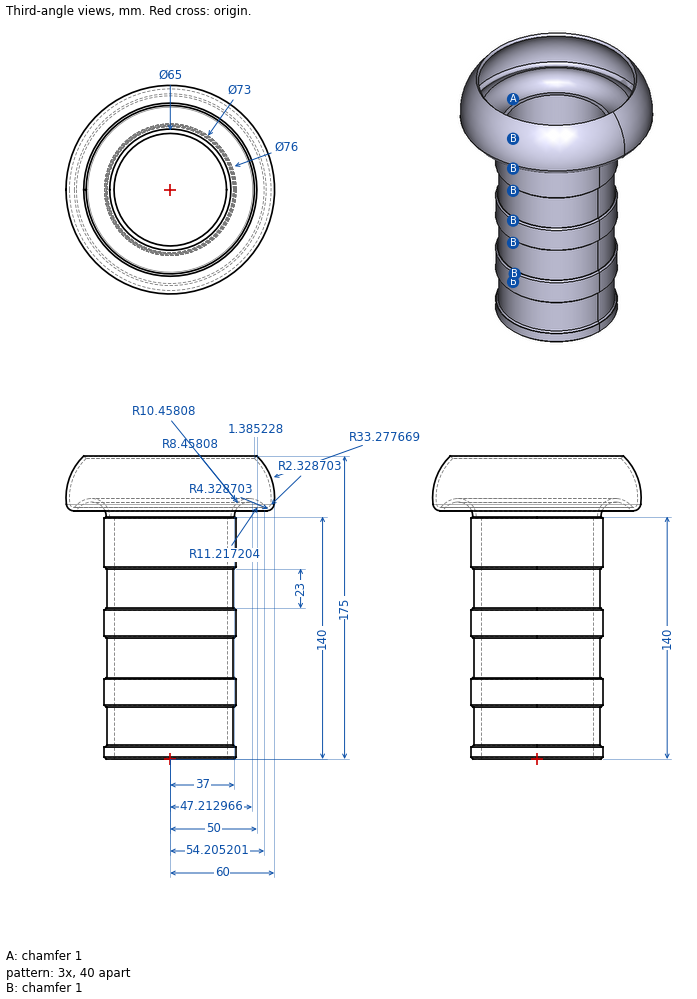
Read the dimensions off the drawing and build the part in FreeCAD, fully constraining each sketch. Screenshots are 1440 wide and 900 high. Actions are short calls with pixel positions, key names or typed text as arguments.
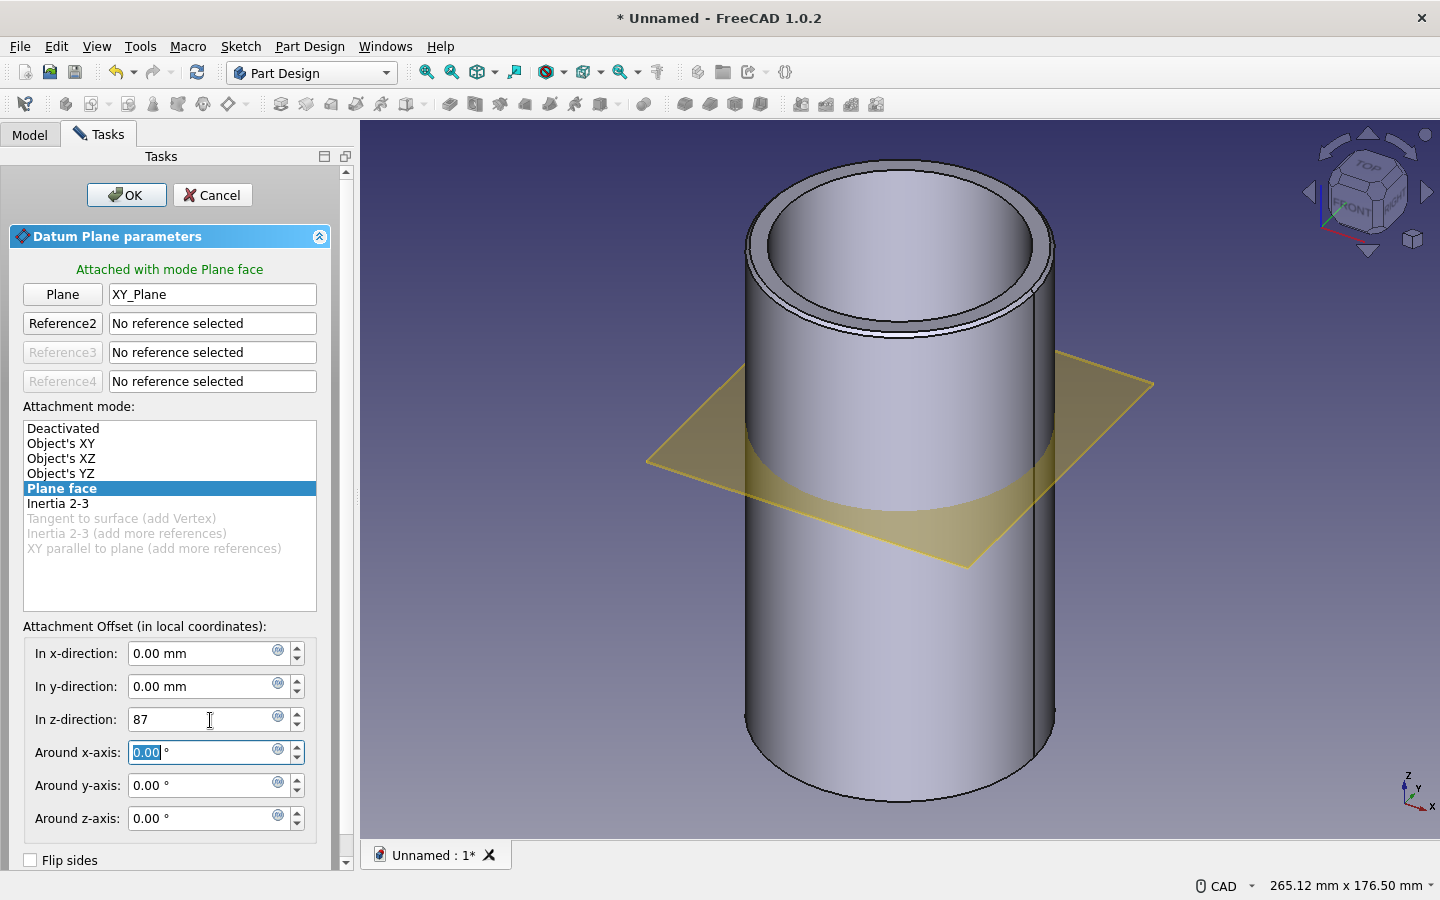
click(127, 195)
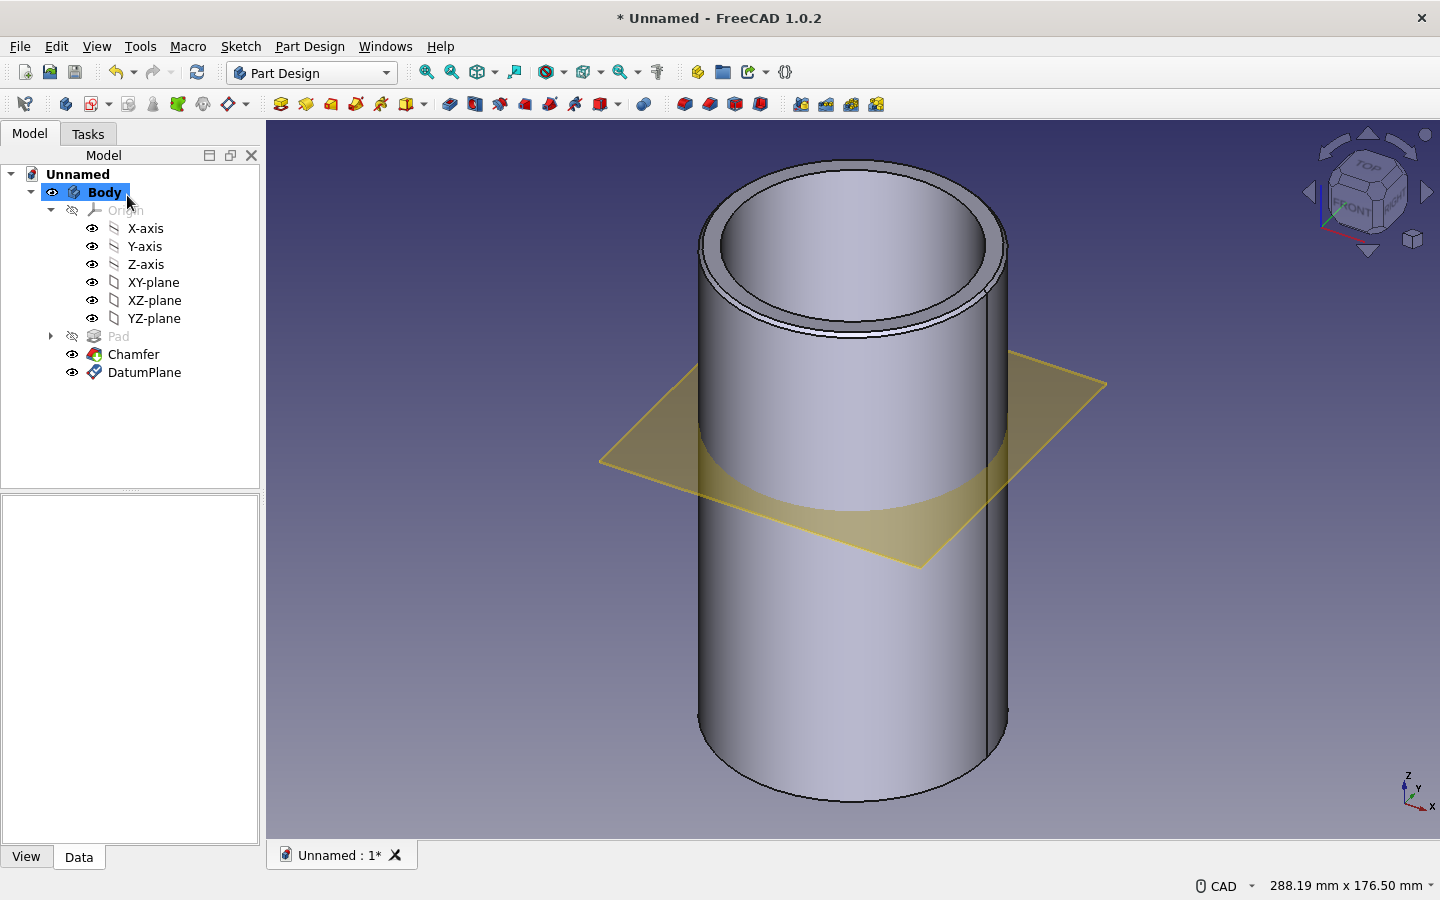
click(117, 372)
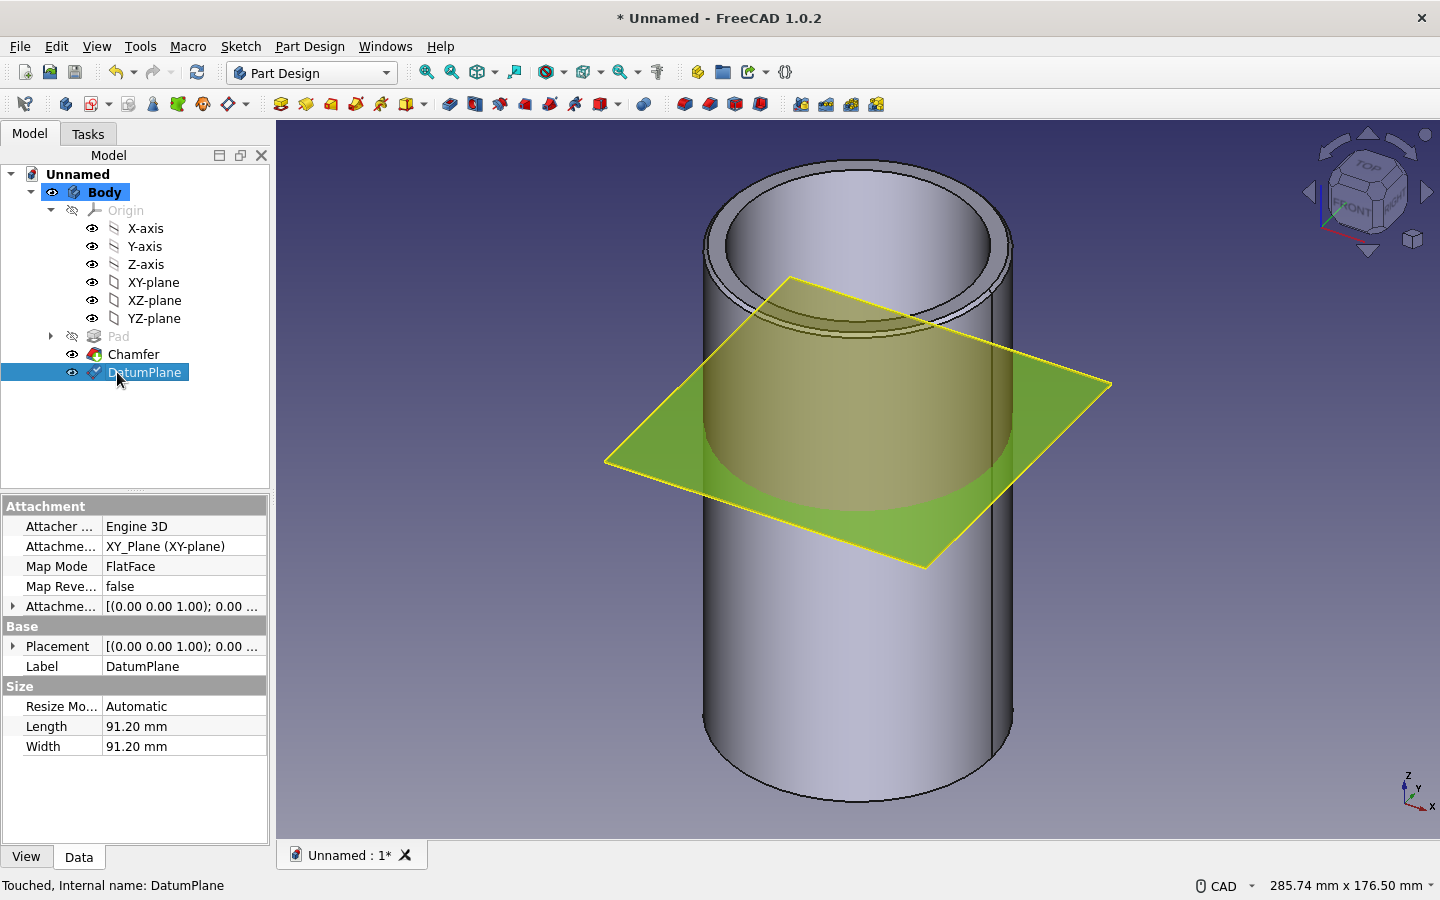
click(90, 104)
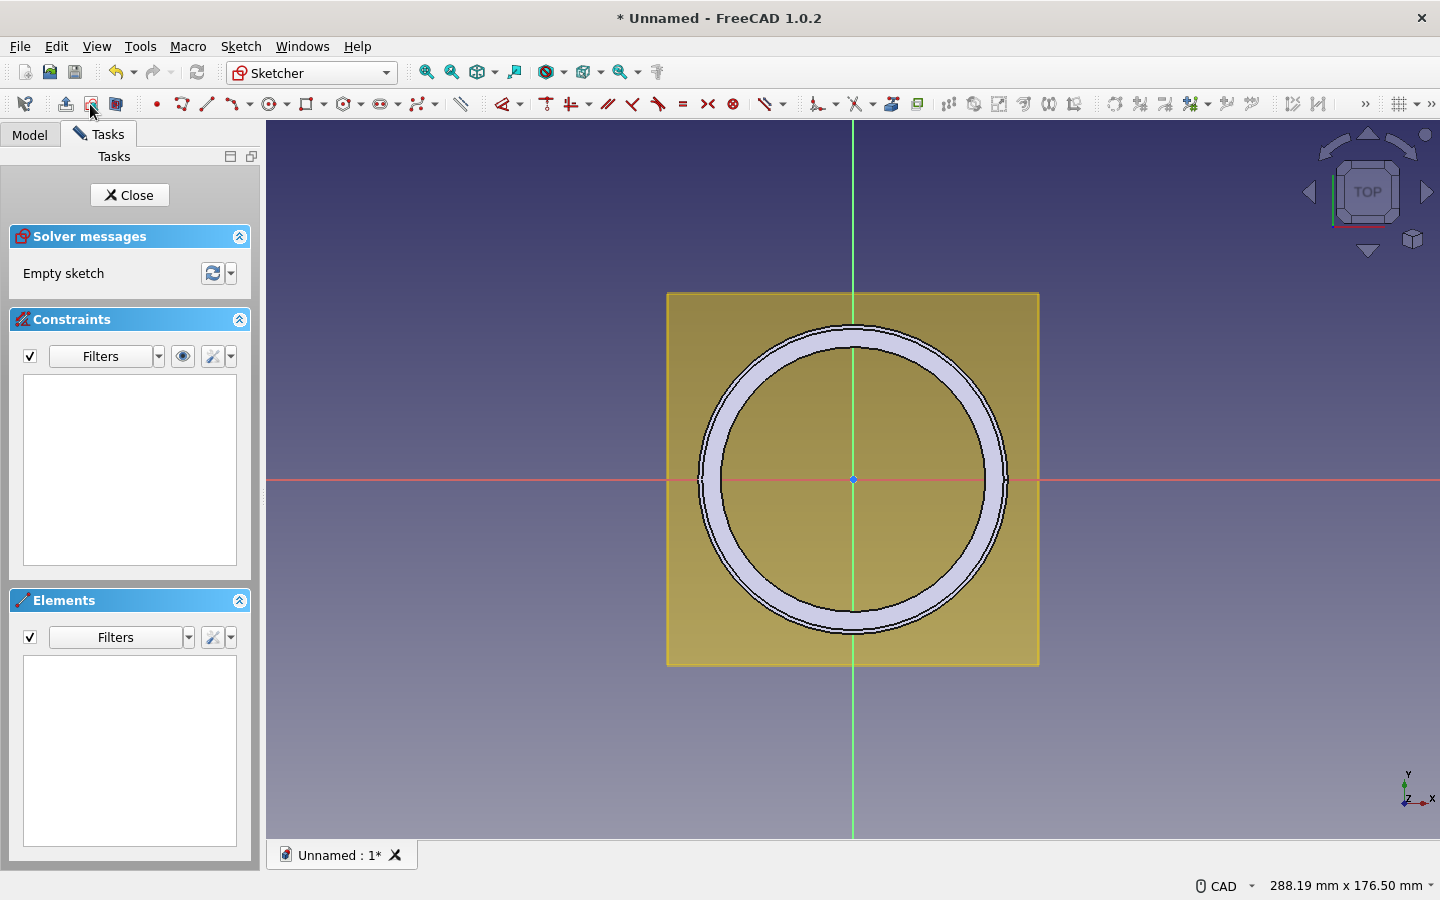
key(q)
key(s)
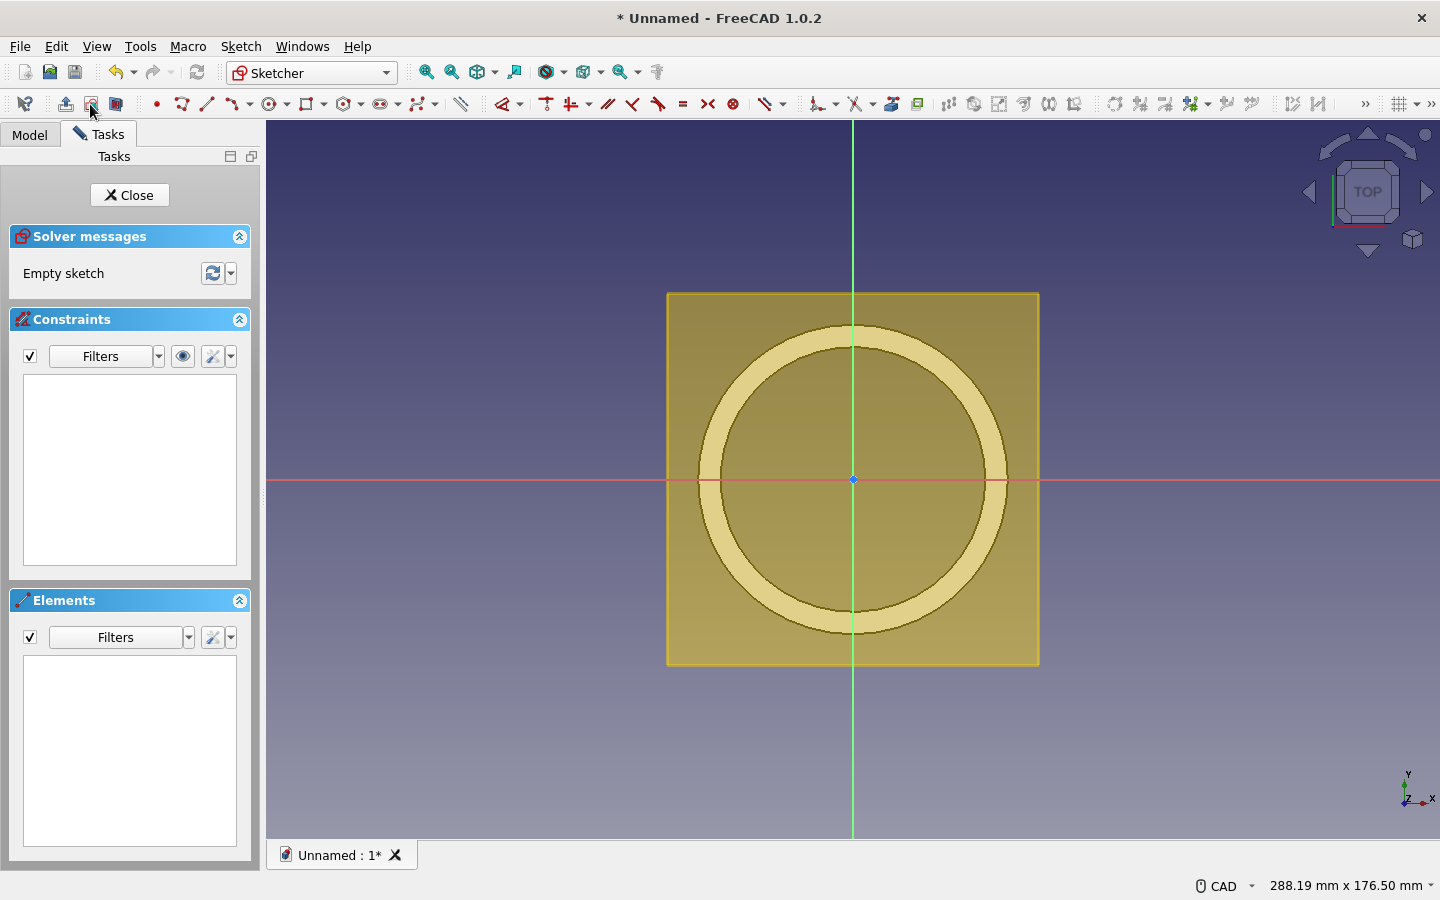
scroll(992, 480, up, 2)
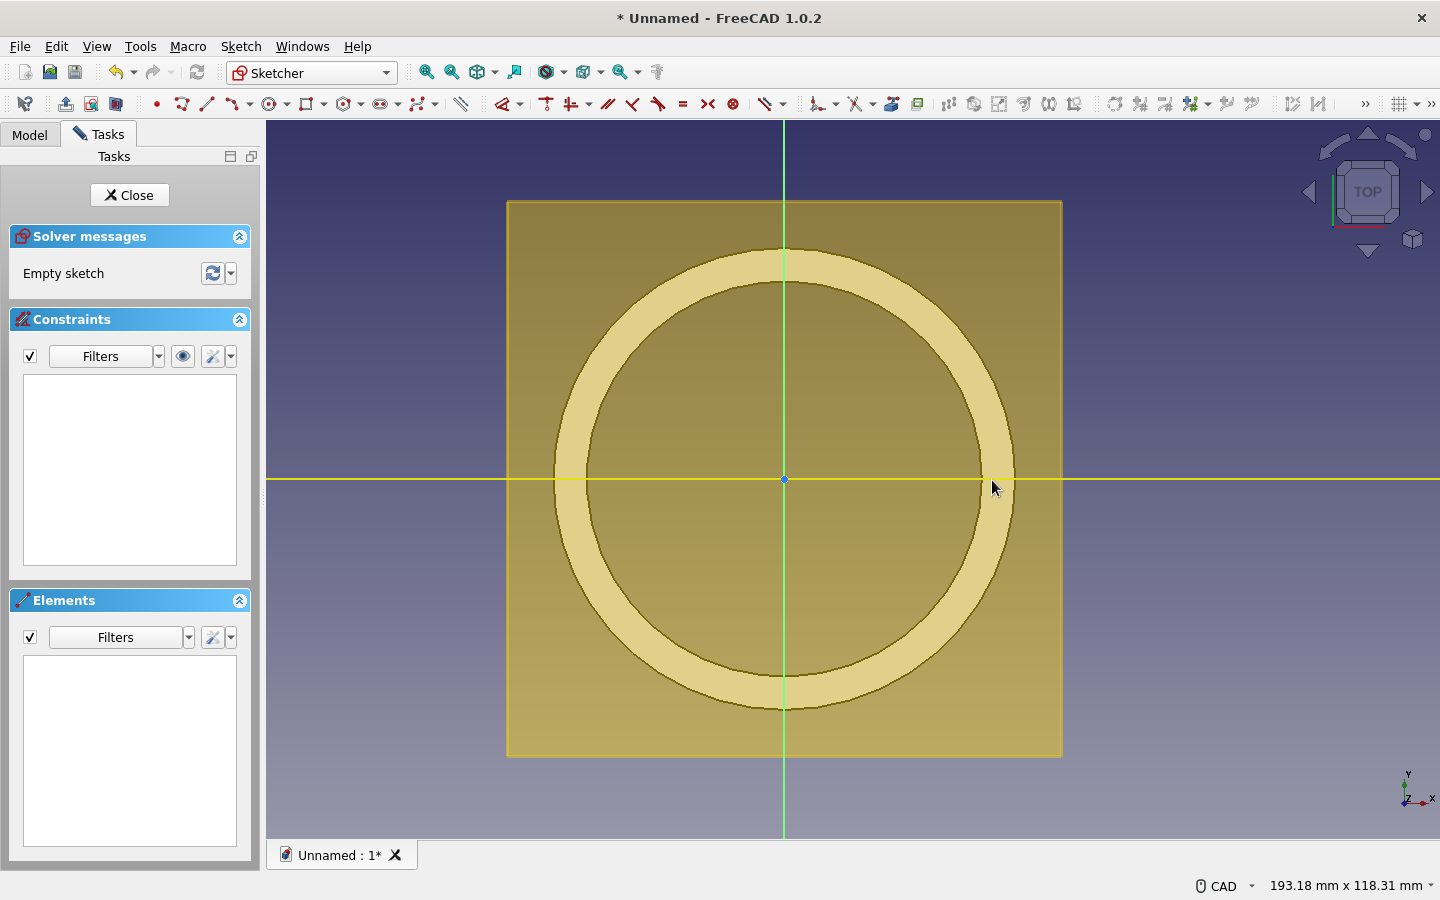
key(g)
key(c)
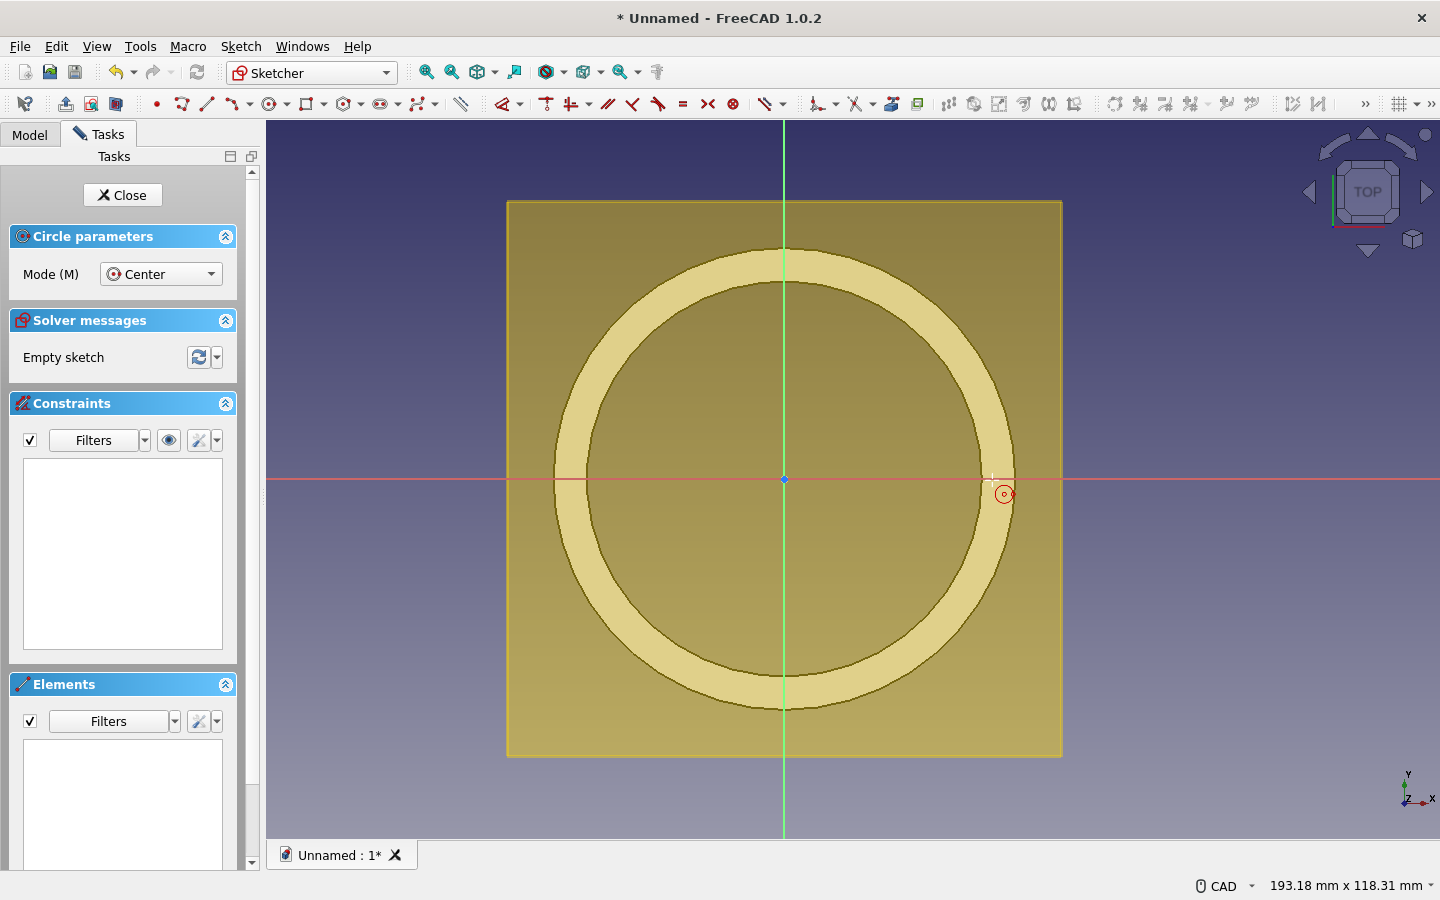
click(784, 479)
move(948, 316)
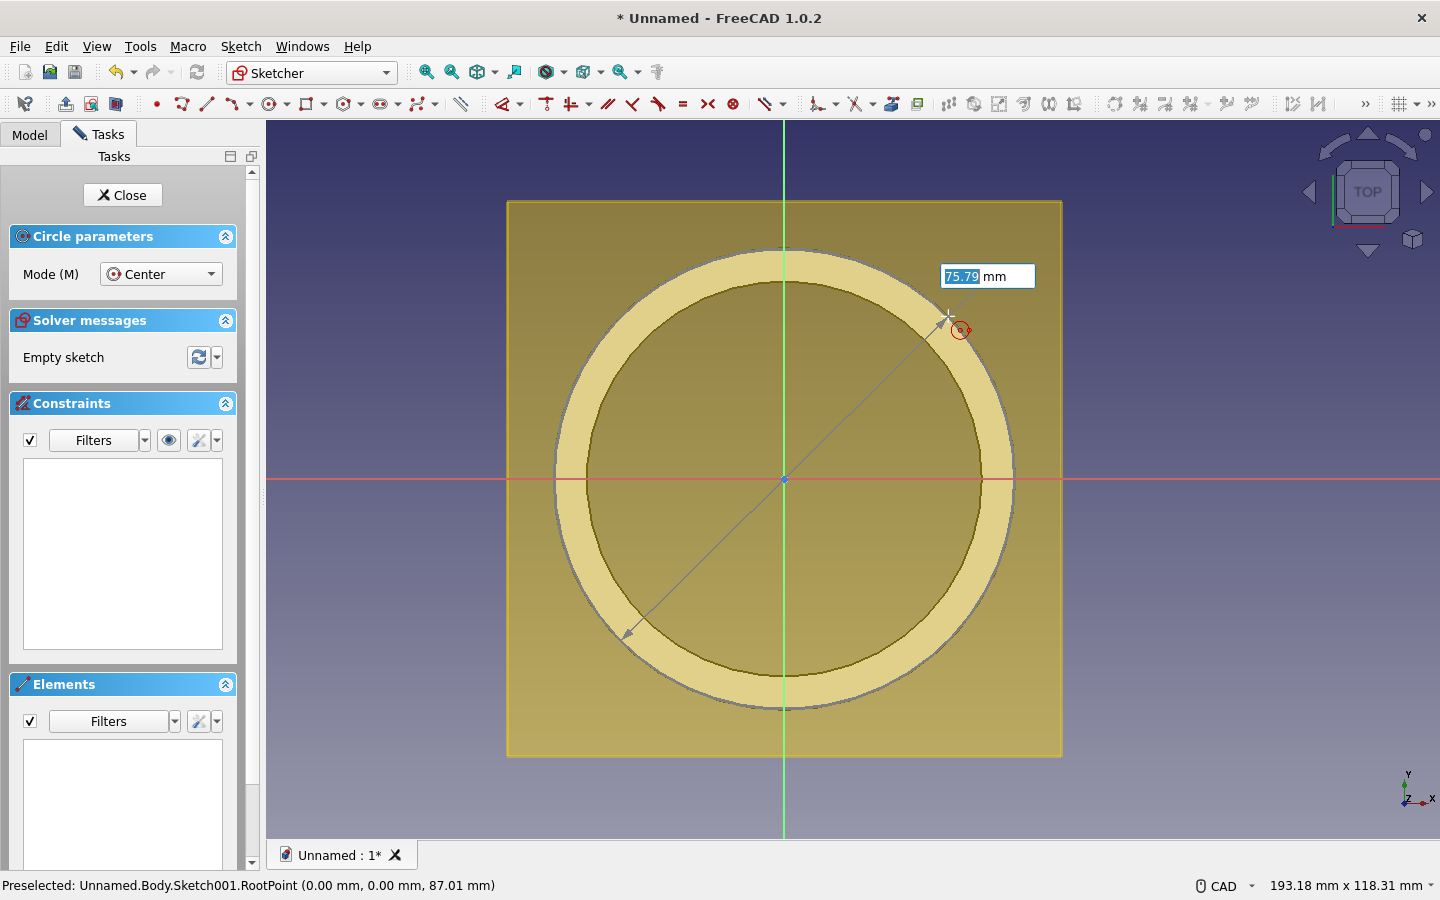
text(76)
key(Return)